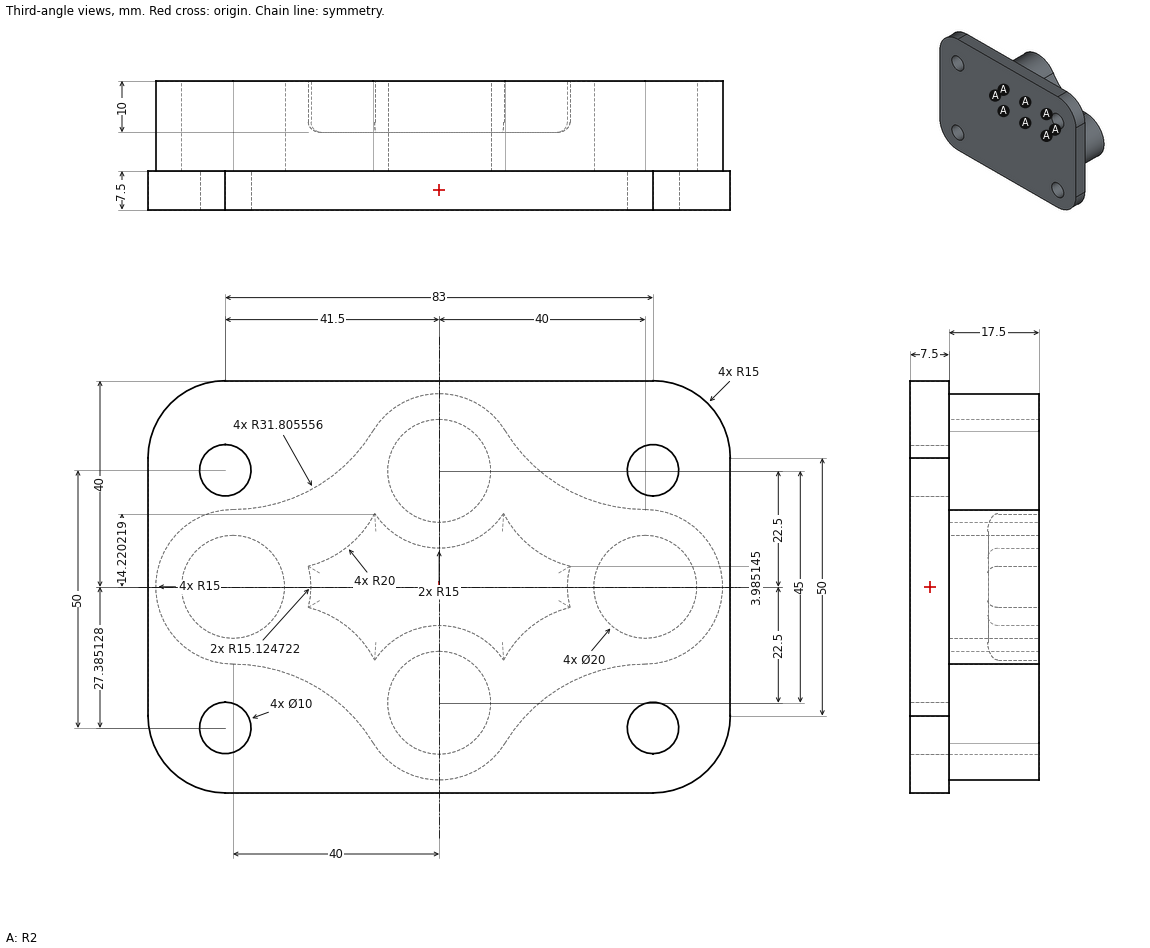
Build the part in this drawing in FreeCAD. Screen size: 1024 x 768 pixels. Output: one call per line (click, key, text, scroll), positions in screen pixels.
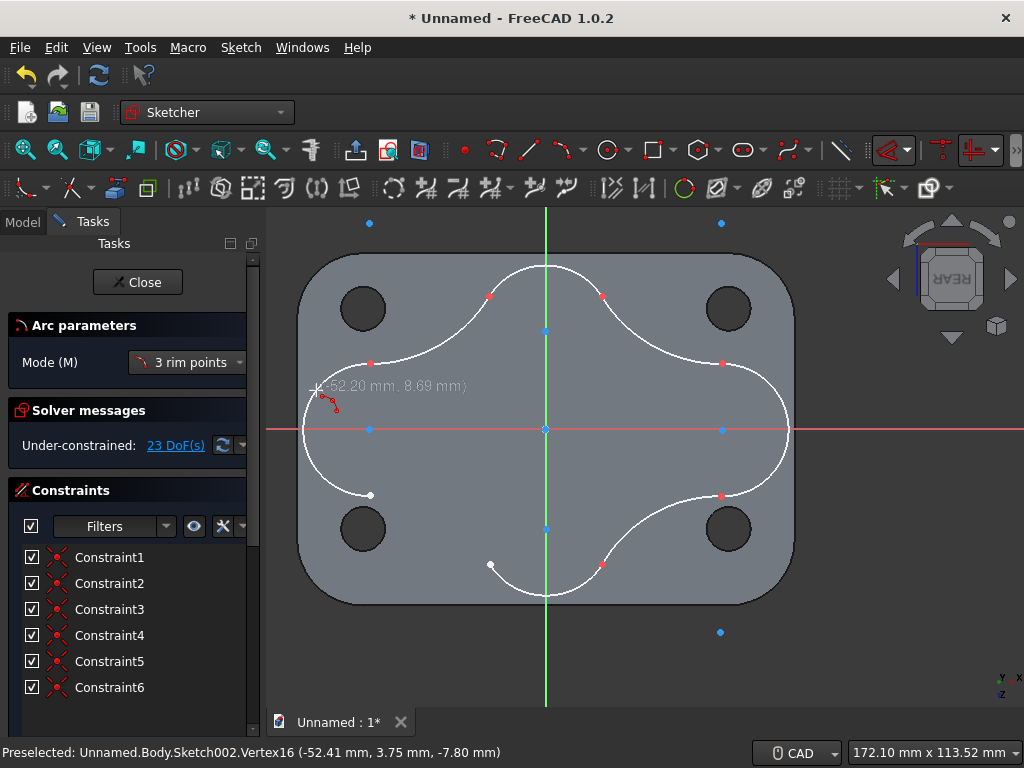
click(370, 496)
click(490, 565)
click(438, 513)
key(Escape)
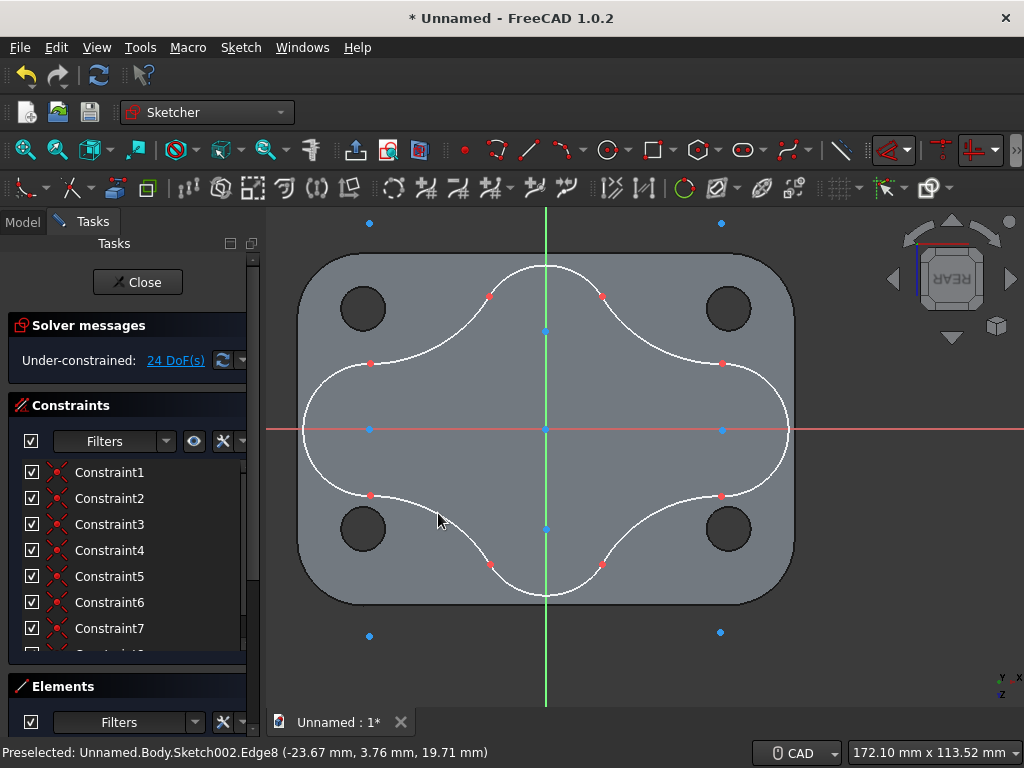
click(520, 590)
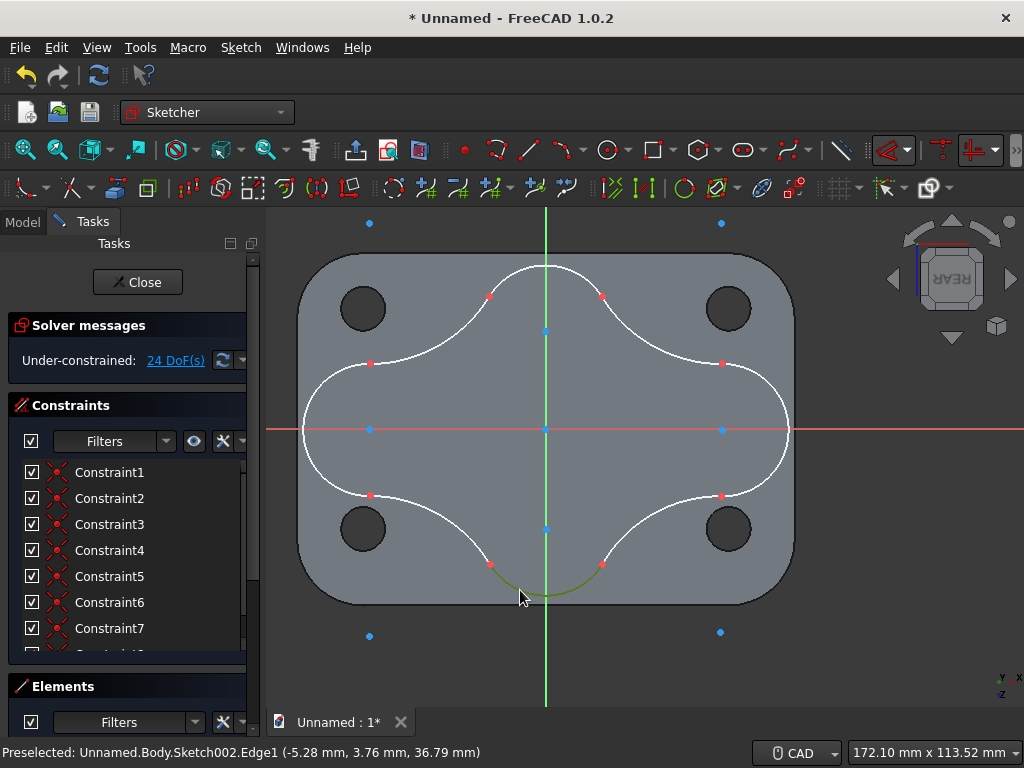
click(679, 503)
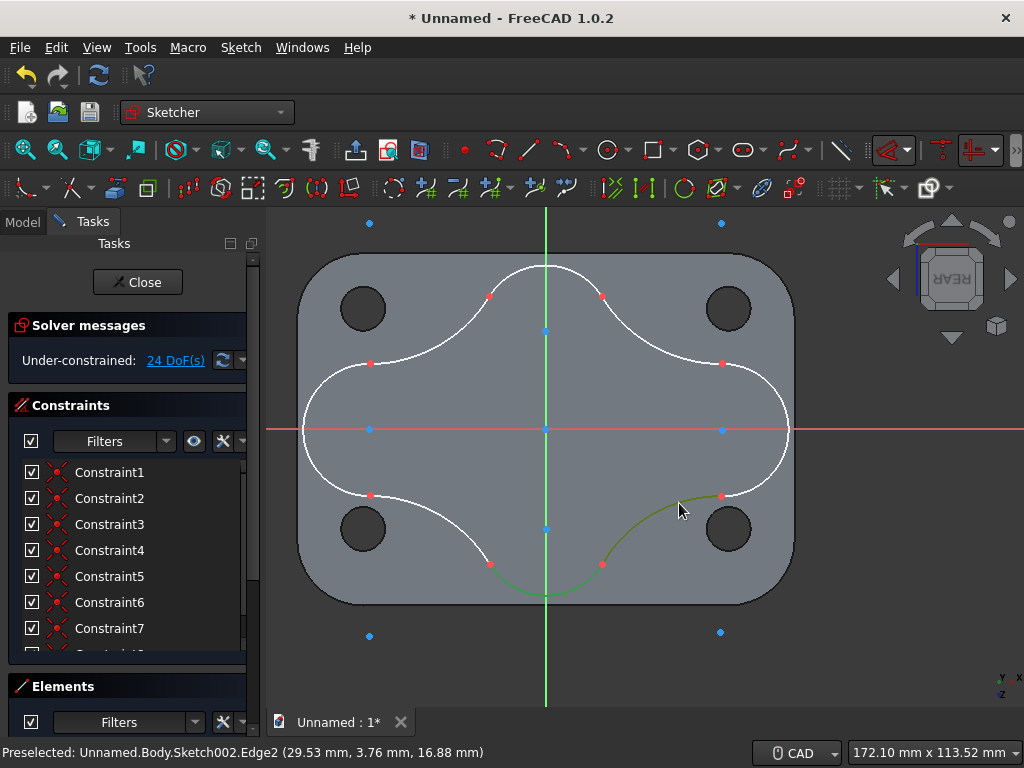
key(t)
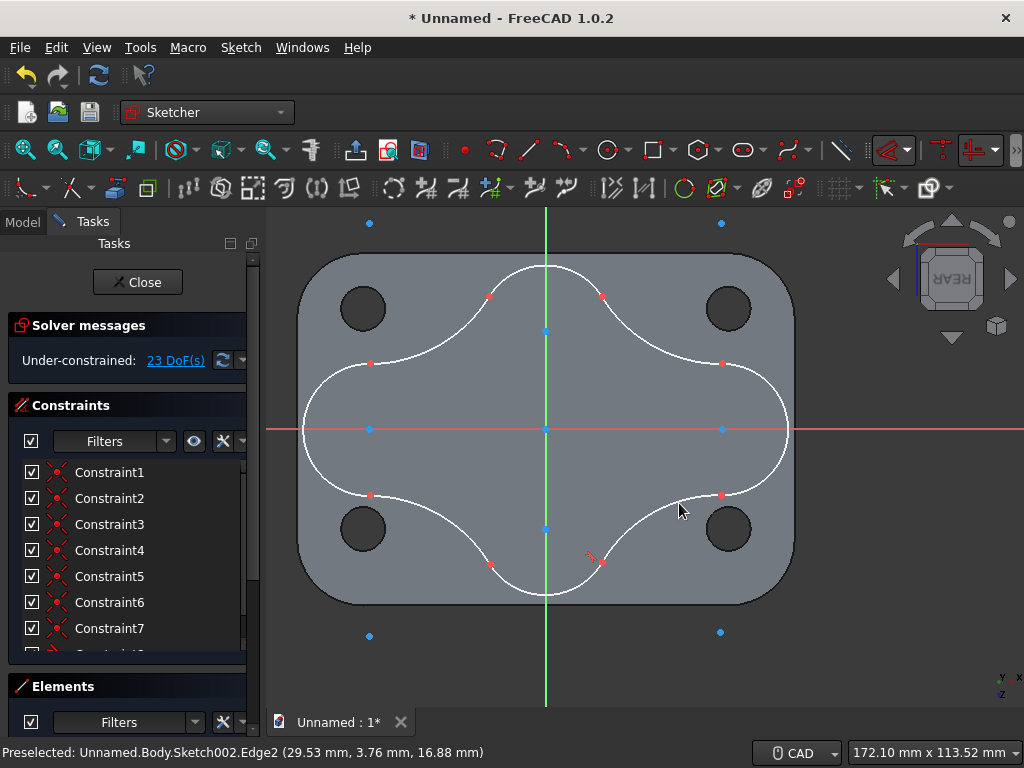
click(521, 590)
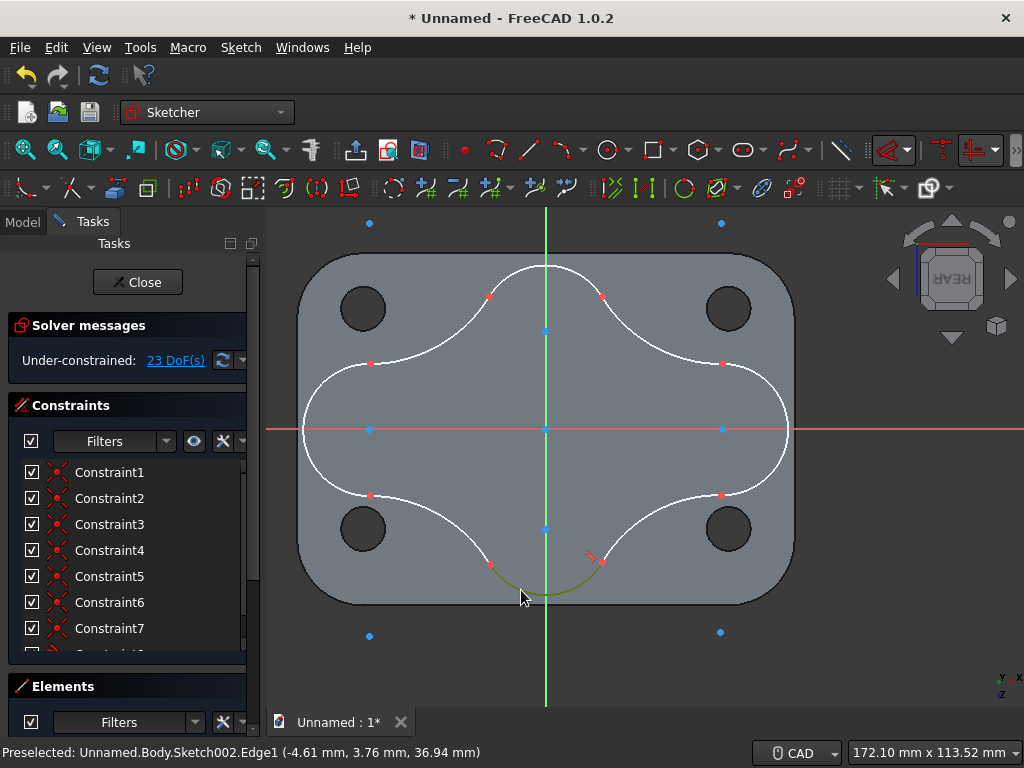
click(463, 532)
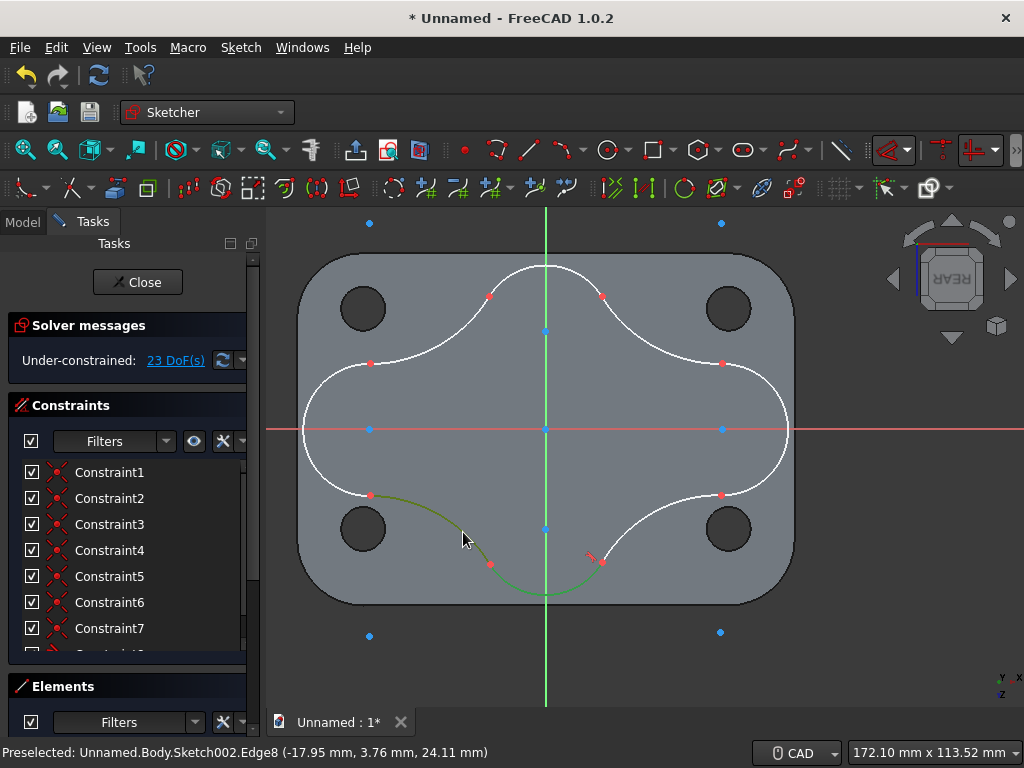
key(t)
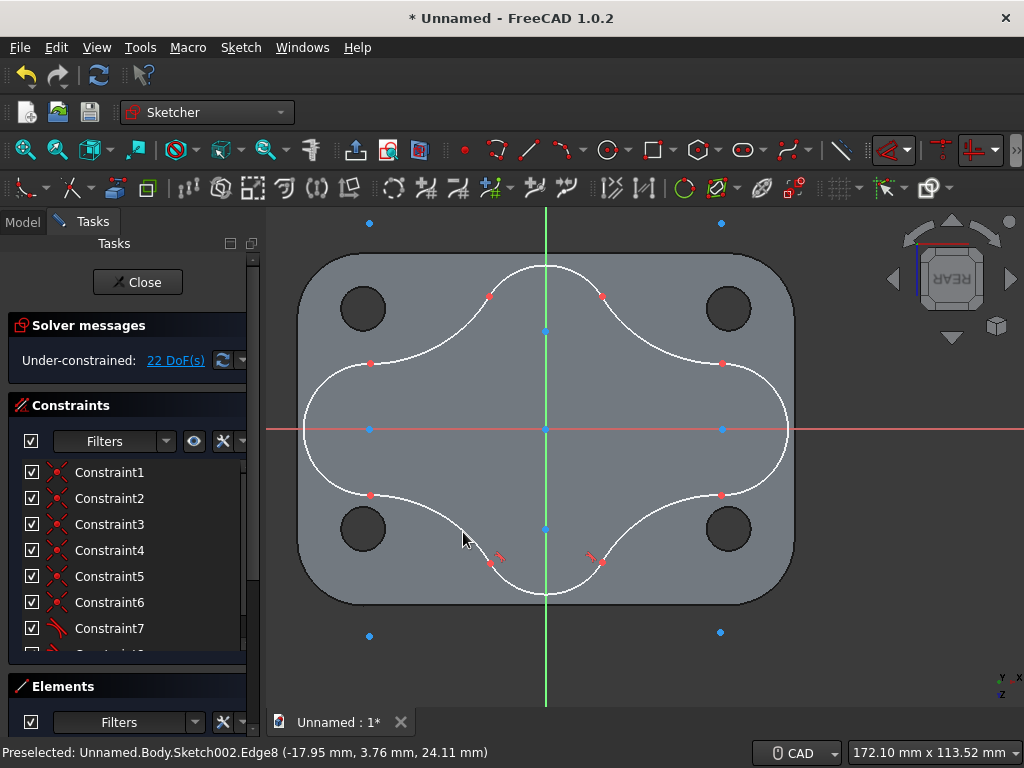
click(679, 501)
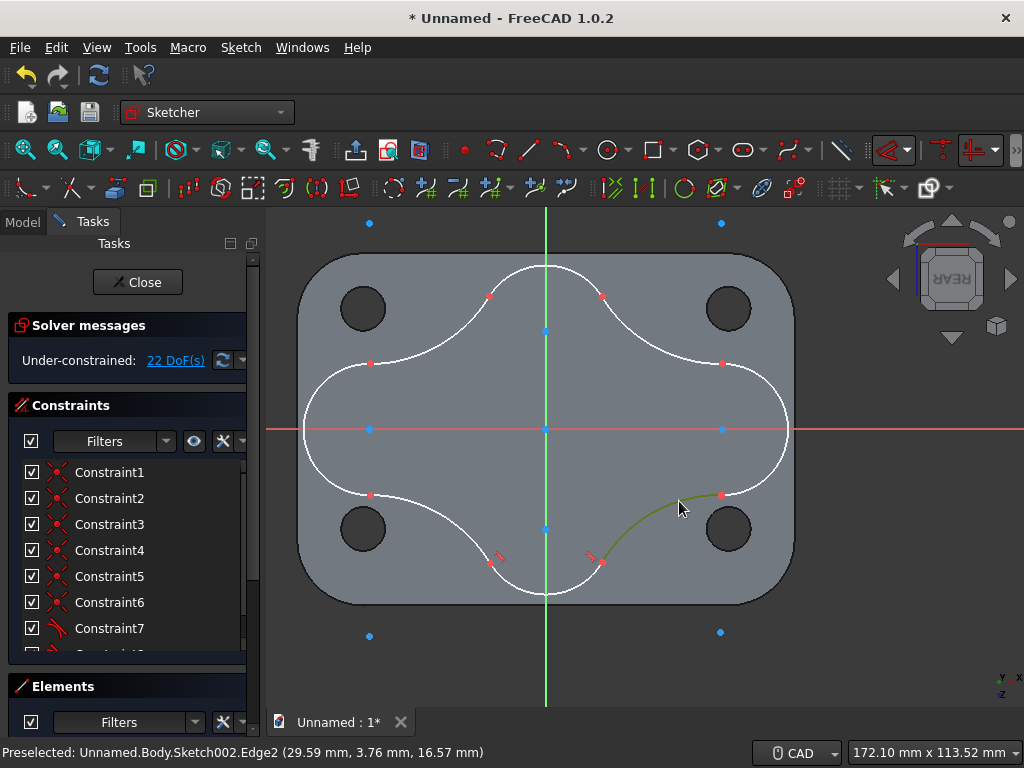
click(775, 469)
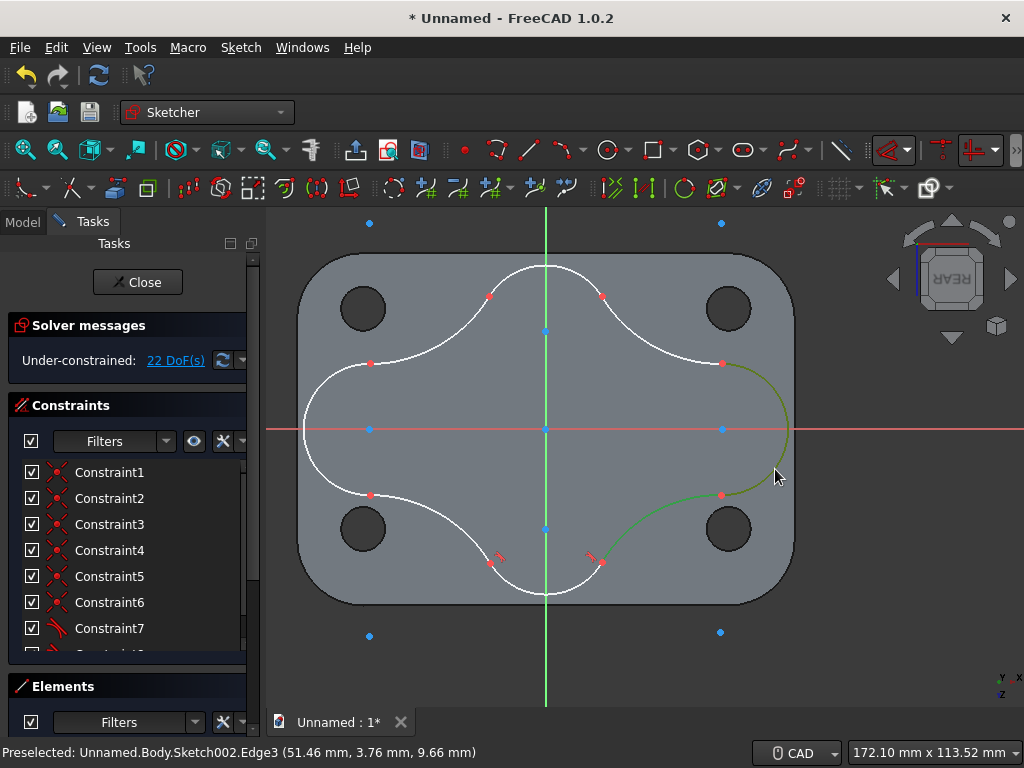
key(t)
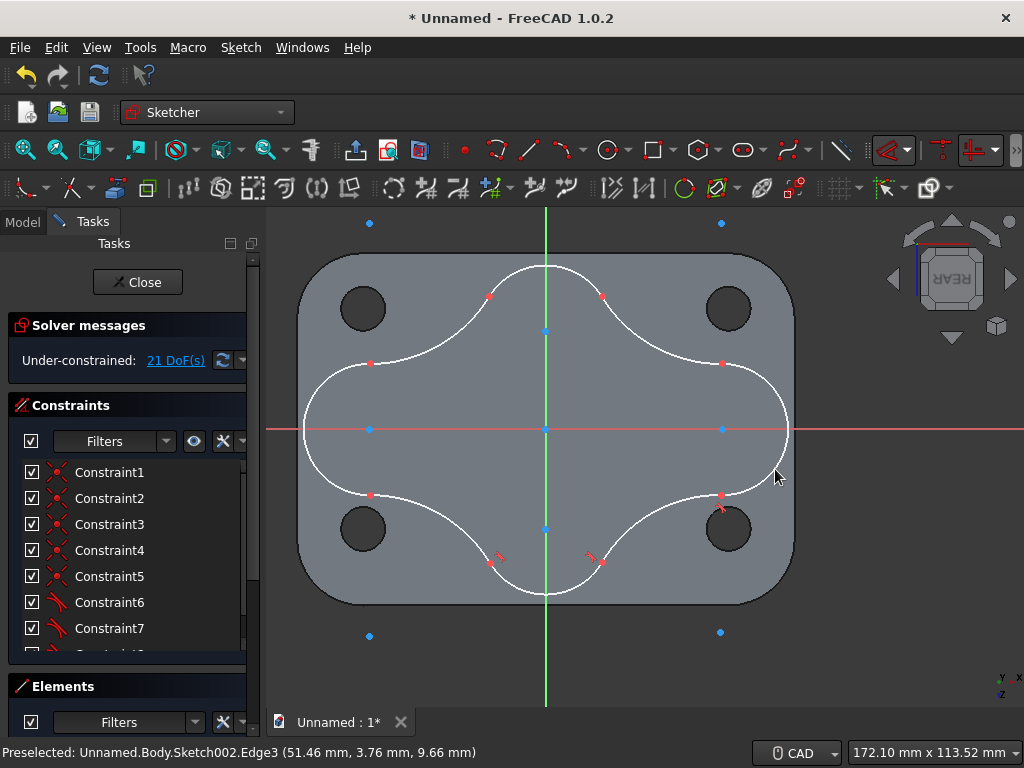
click(775, 468)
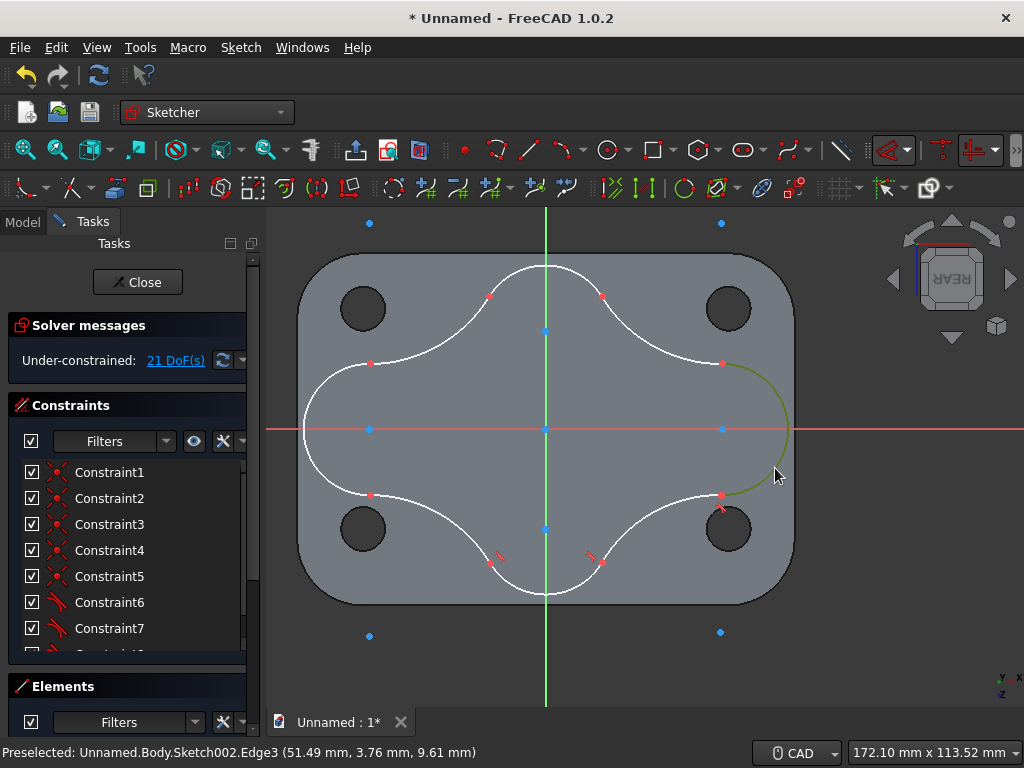
click(630, 330)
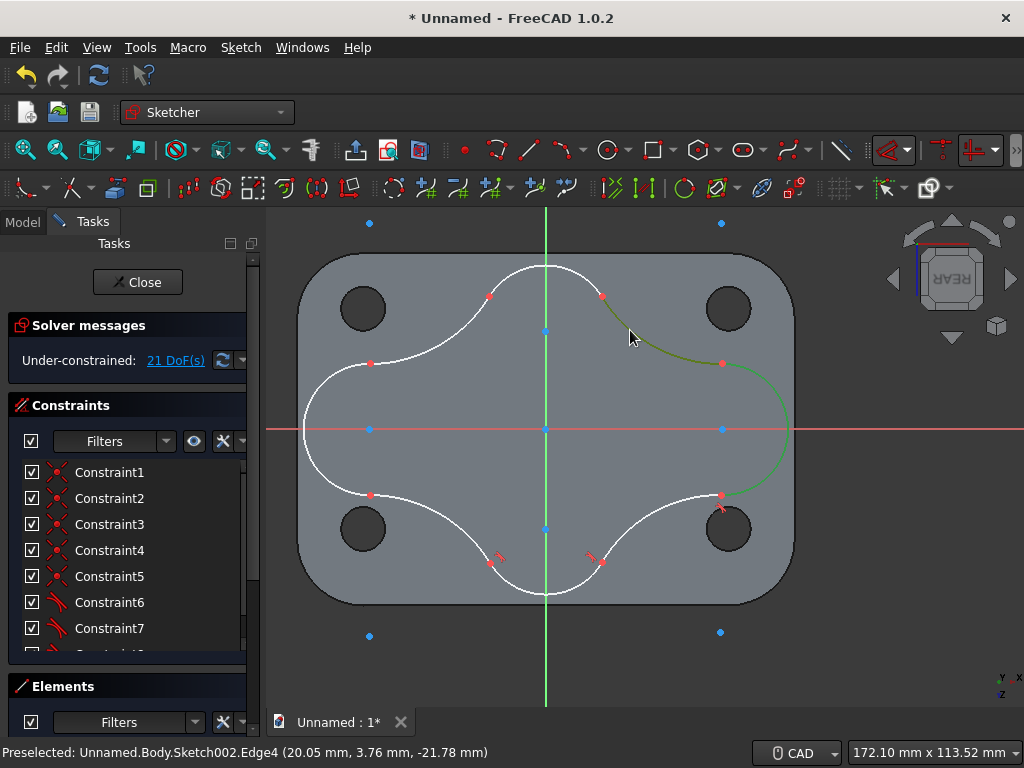
key(t)